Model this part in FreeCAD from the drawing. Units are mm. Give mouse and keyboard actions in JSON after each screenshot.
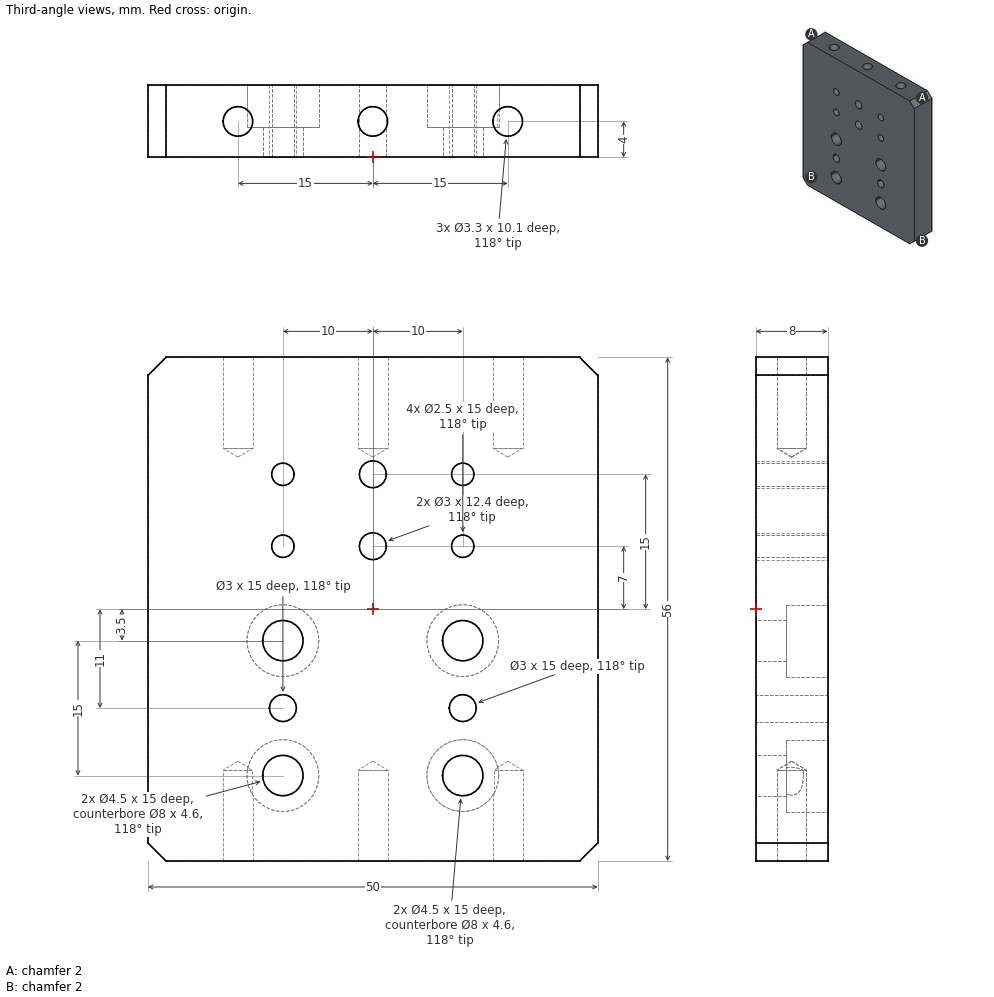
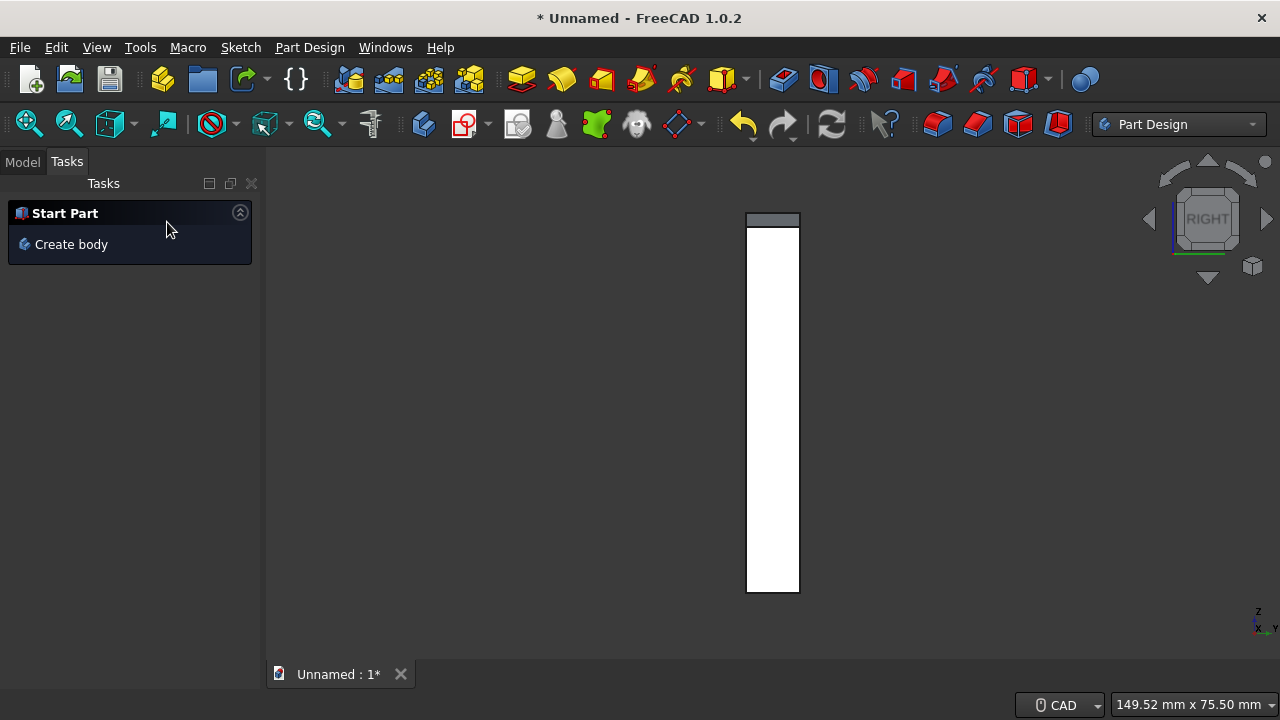
{"action": "left_click", "coordinate": [773, 592]}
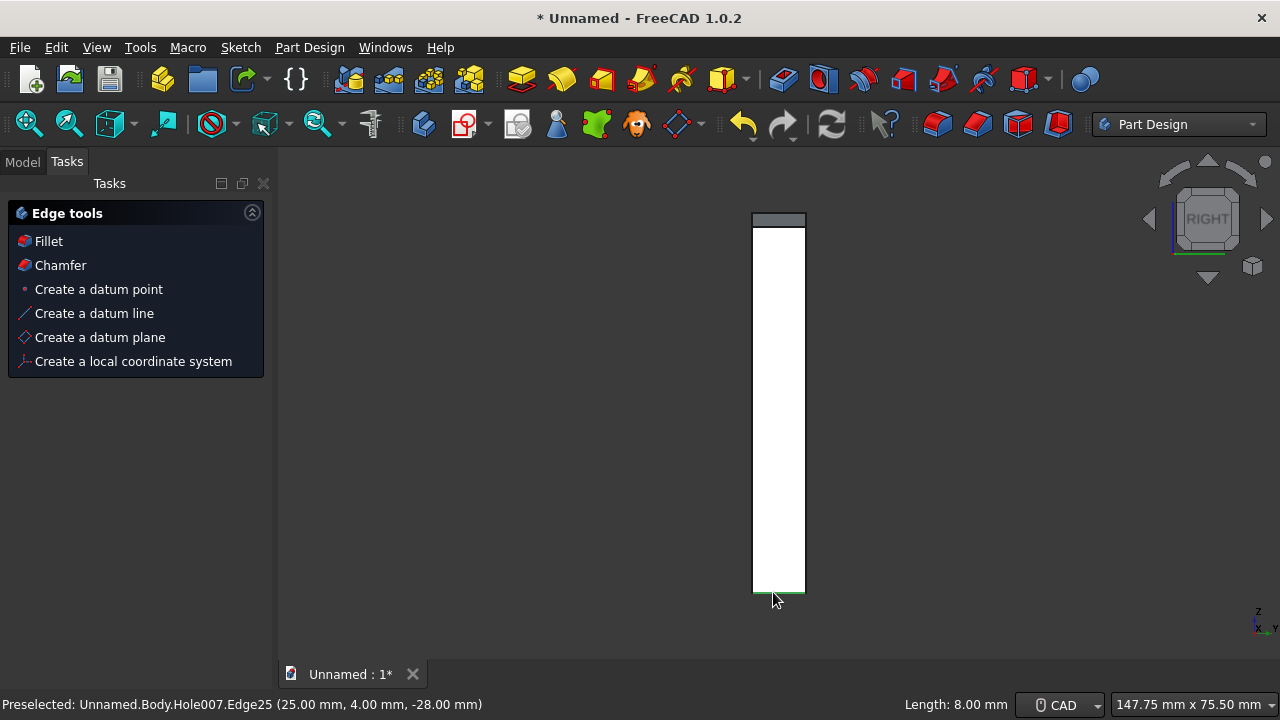
{"action": "key", "text": "5"}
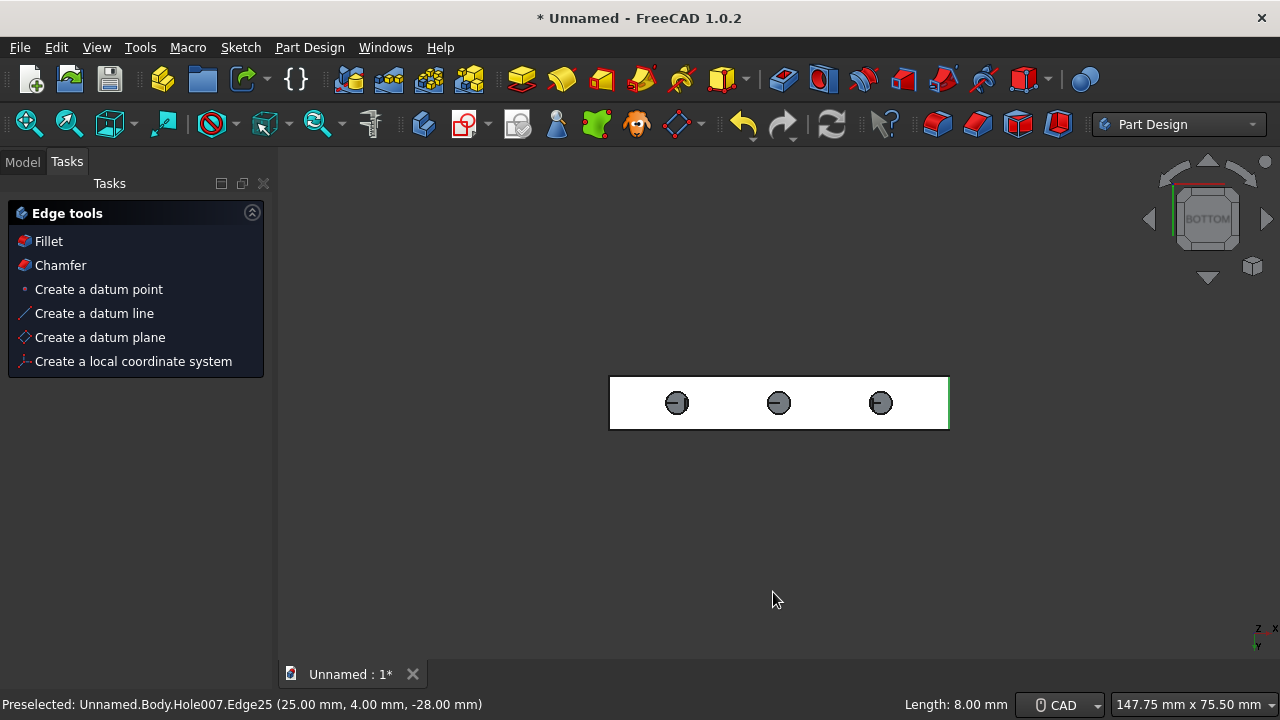
{"action": "left_click", "coordinate": [30, 124]}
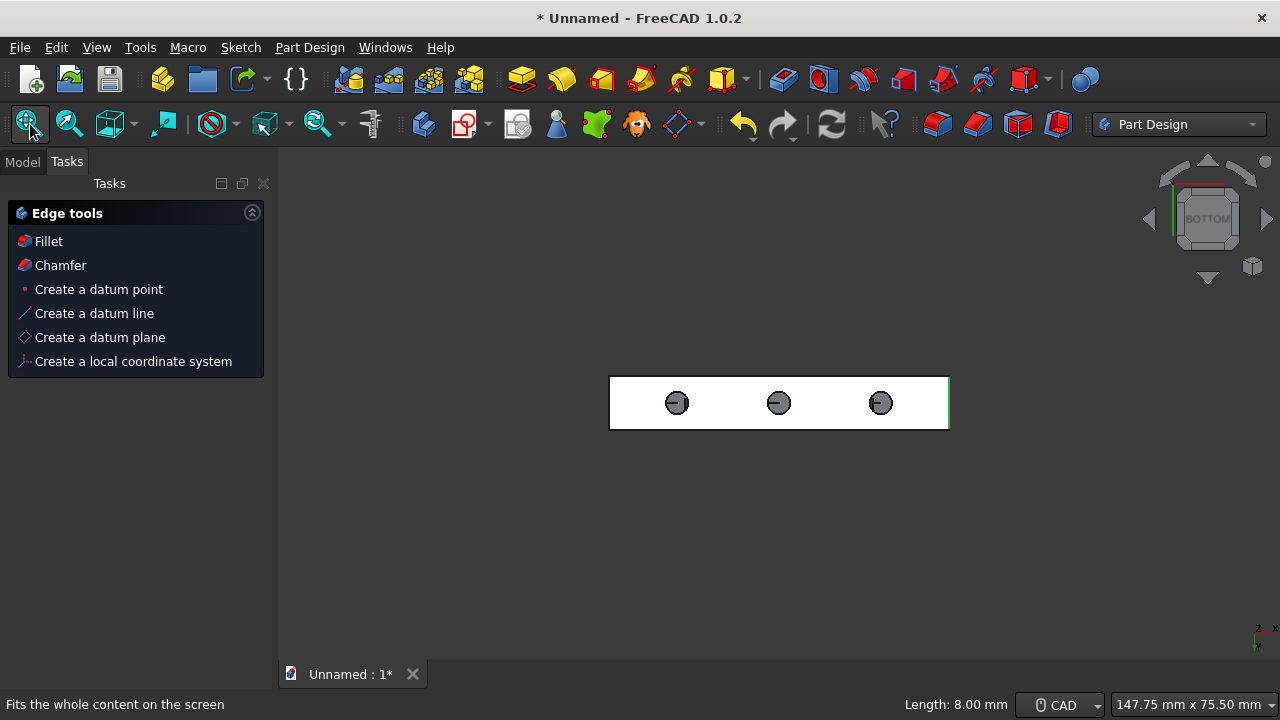
{"action": "left_click", "coordinate": [609, 402], "text": "ctrl"}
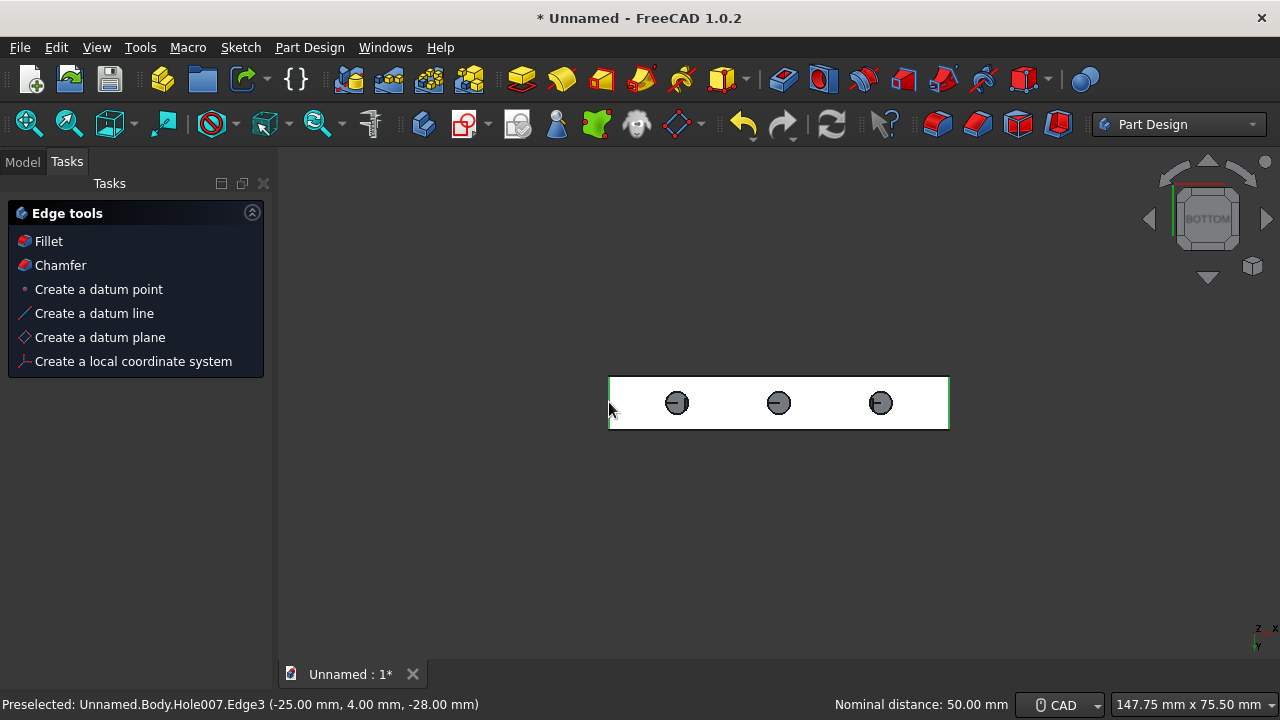
{"action": "left_click", "coordinate": [978, 124]}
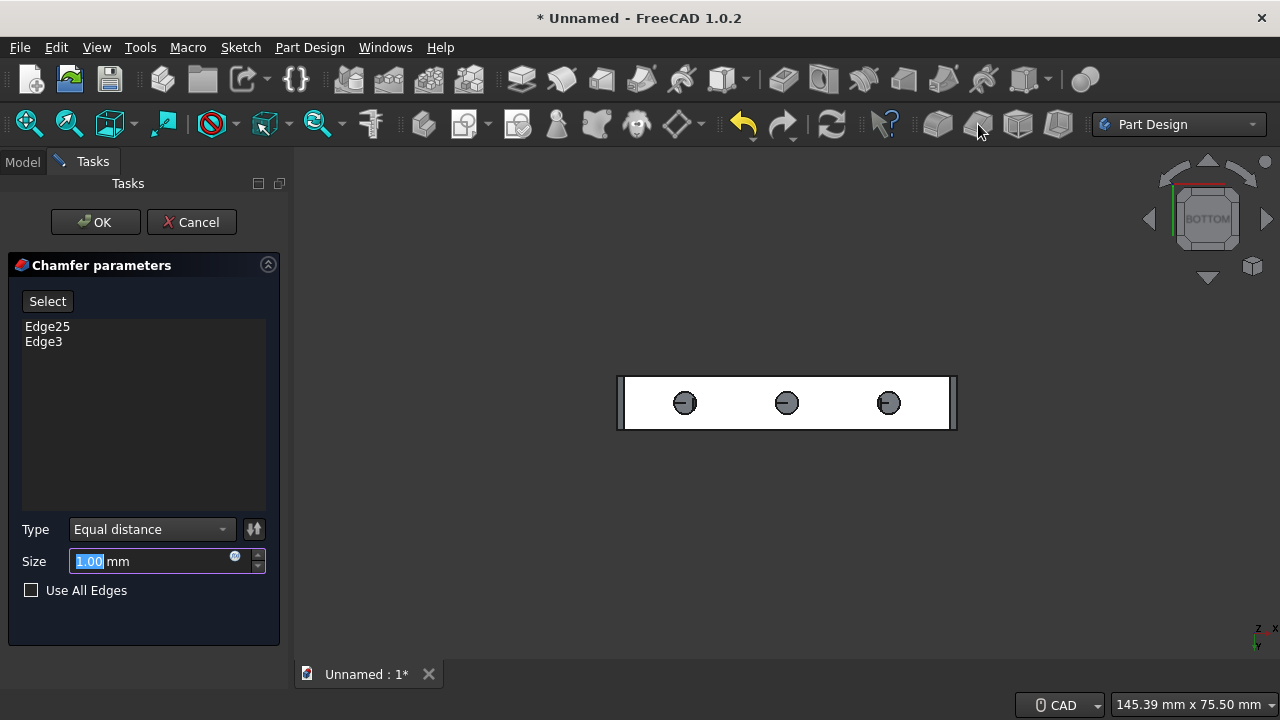
{"action": "type", "text": "2"}
{"action": "key", "text": "Tab"}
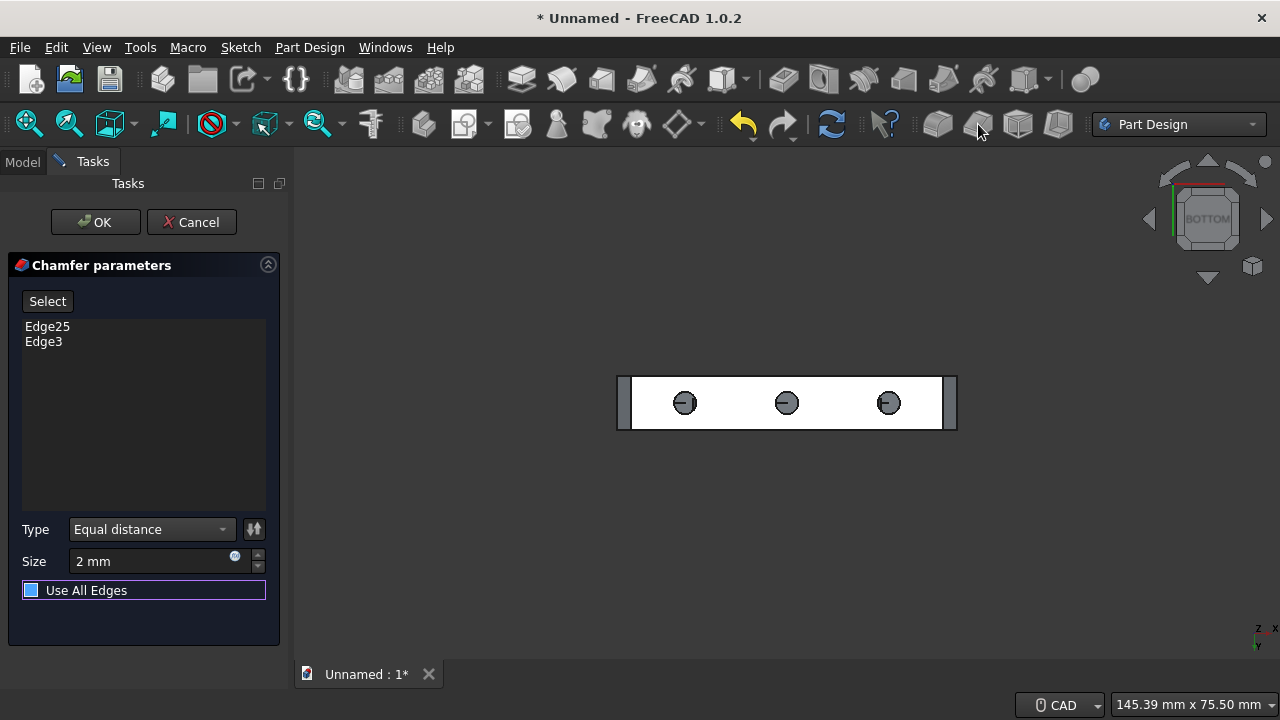
{"action": "left_click", "coordinate": [96, 222]}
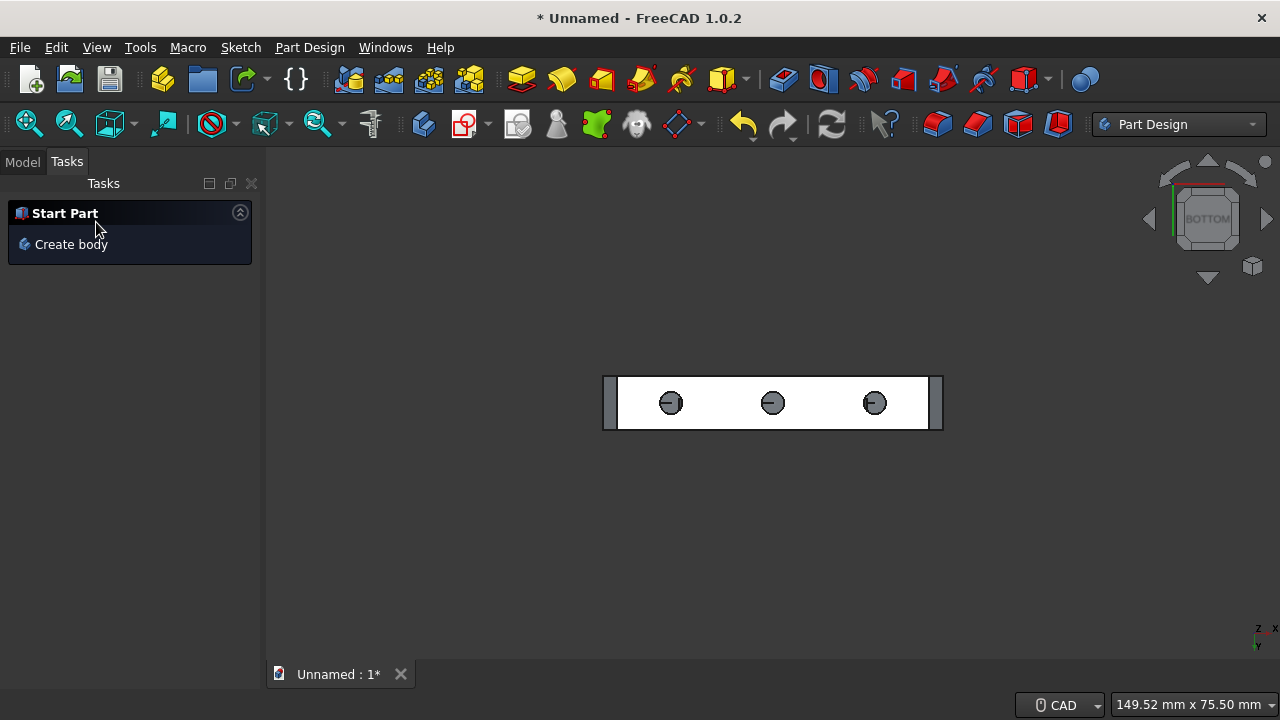
{"action": "key", "text": "0"}